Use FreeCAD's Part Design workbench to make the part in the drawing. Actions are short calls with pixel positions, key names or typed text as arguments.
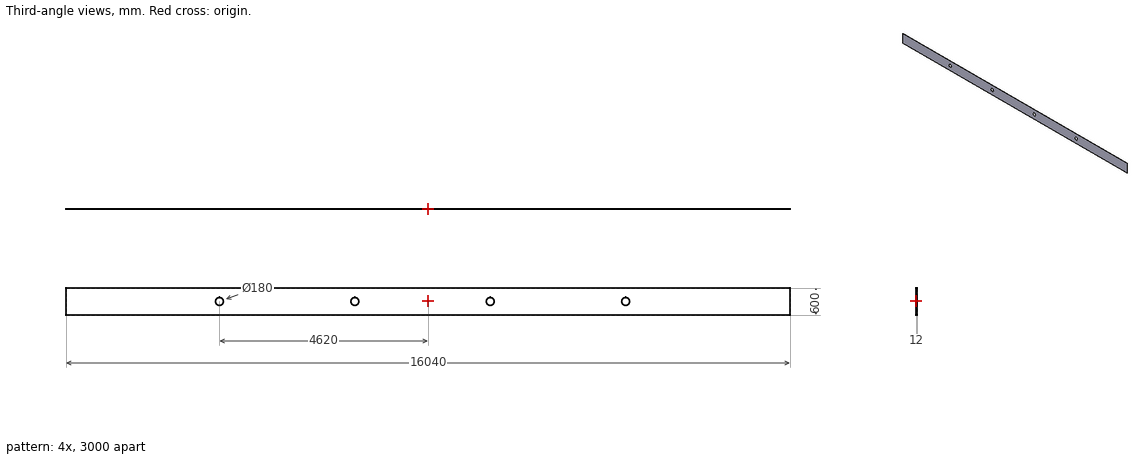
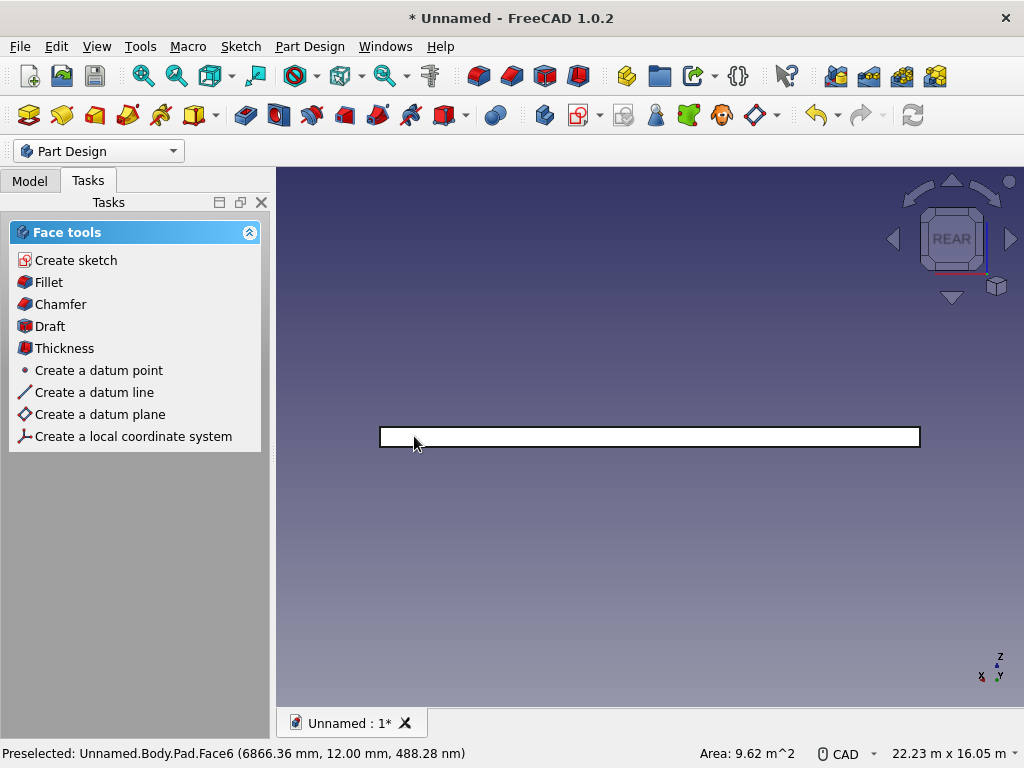
click(578, 116)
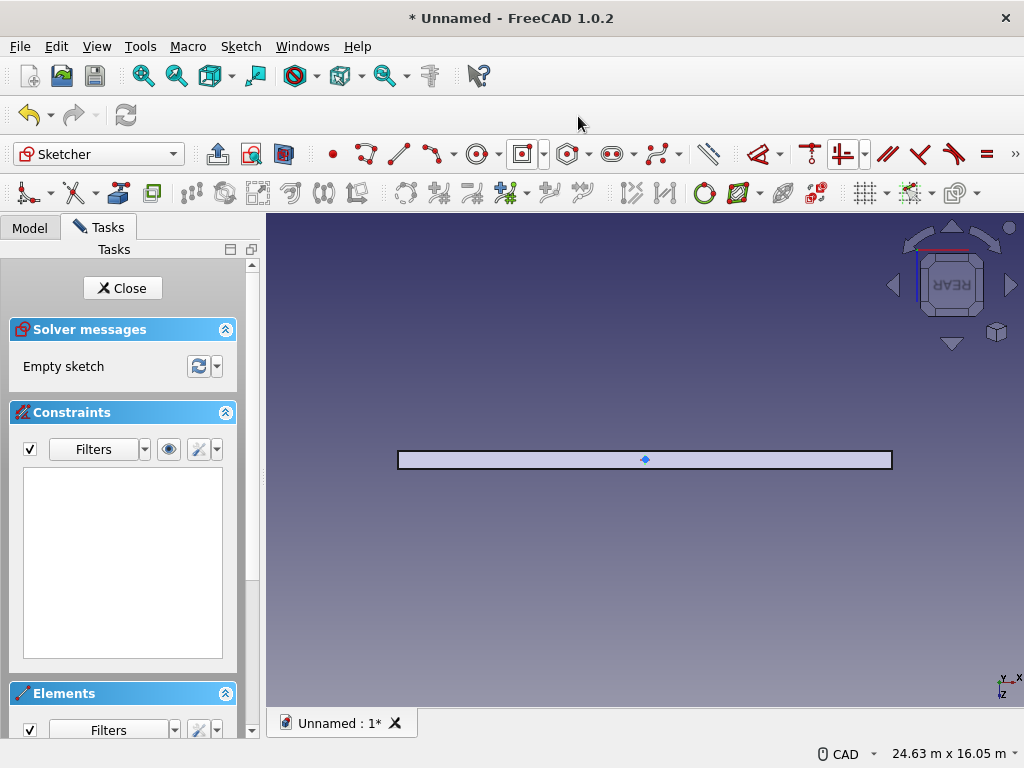
scroll(499, 460, up, 15)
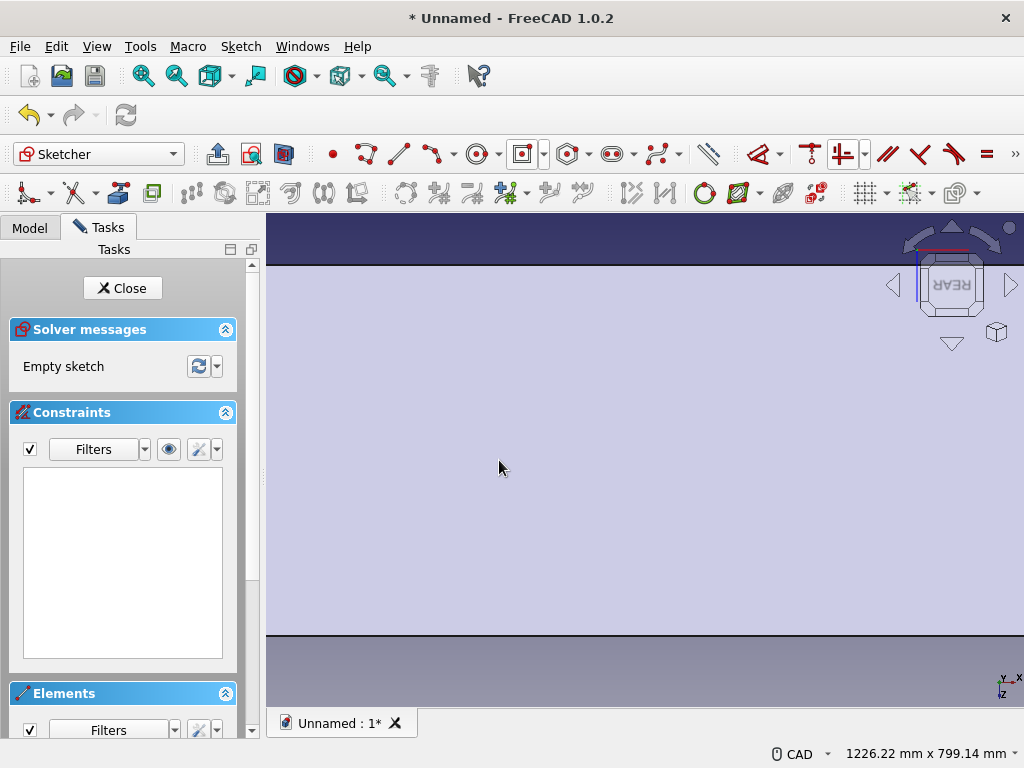
scroll(566, 445, up, 5)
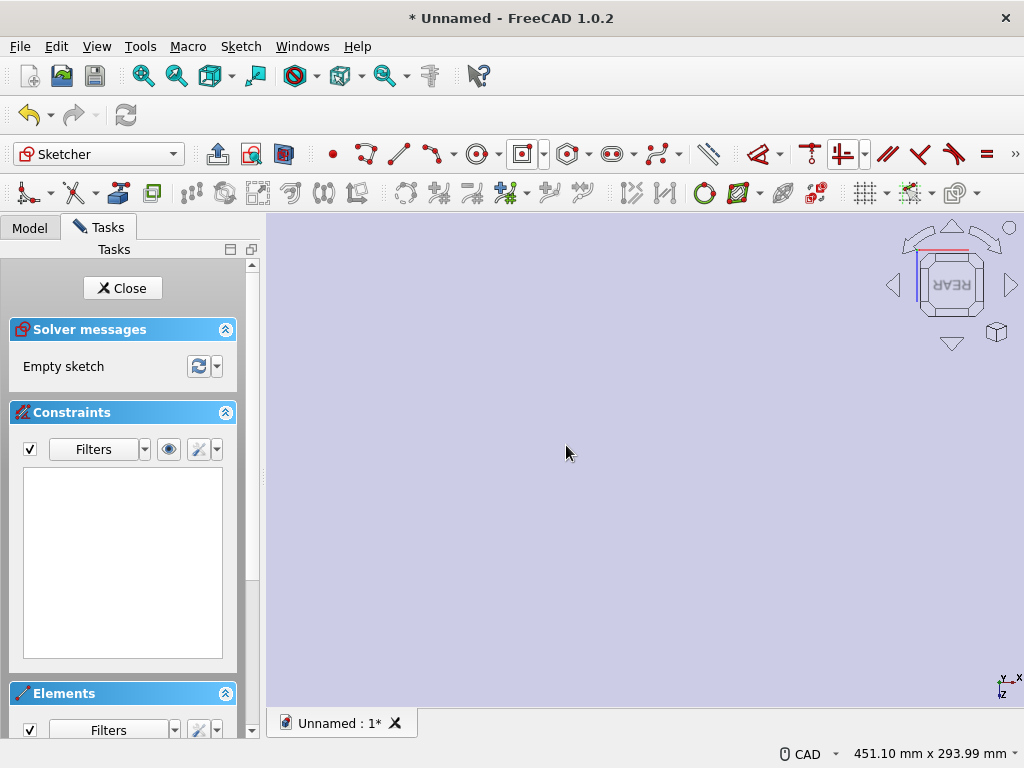
click(476, 154)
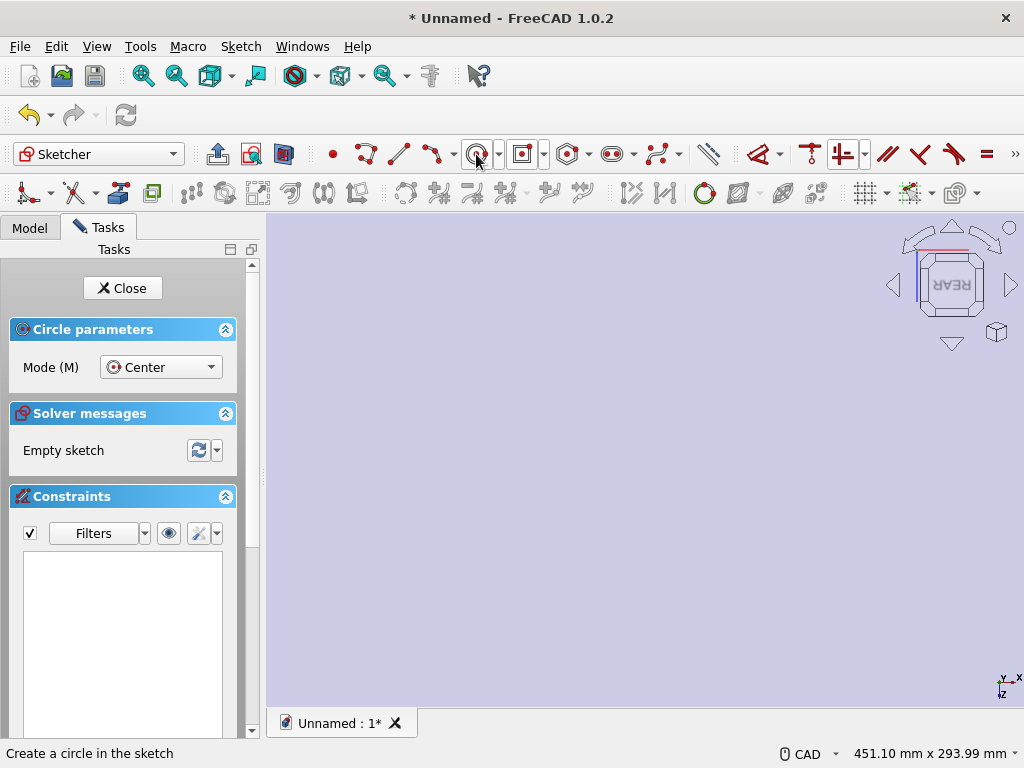
click(575, 459)
move(682, 352)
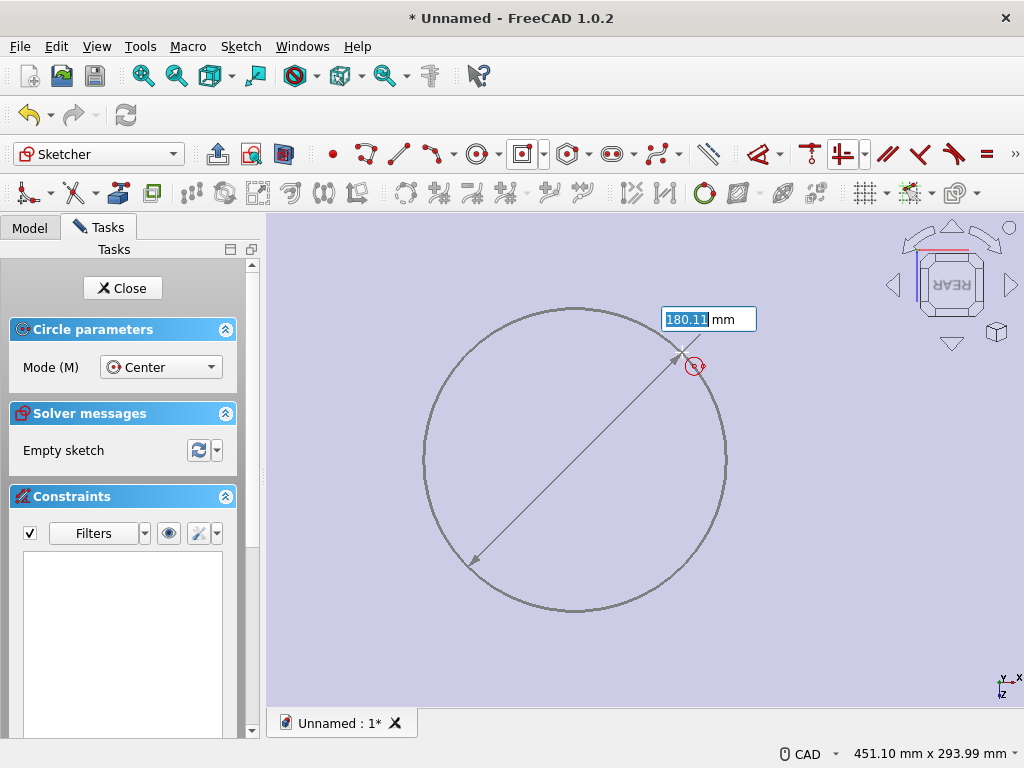
text(180)
key(Return)
key(Escape)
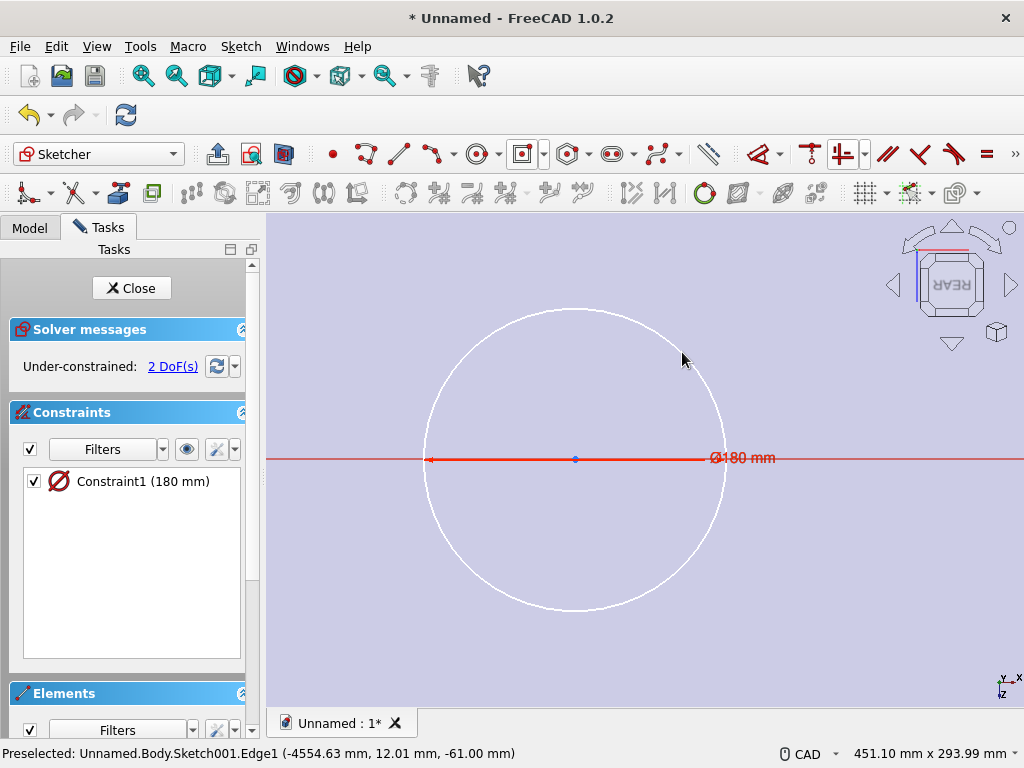
click(575, 460)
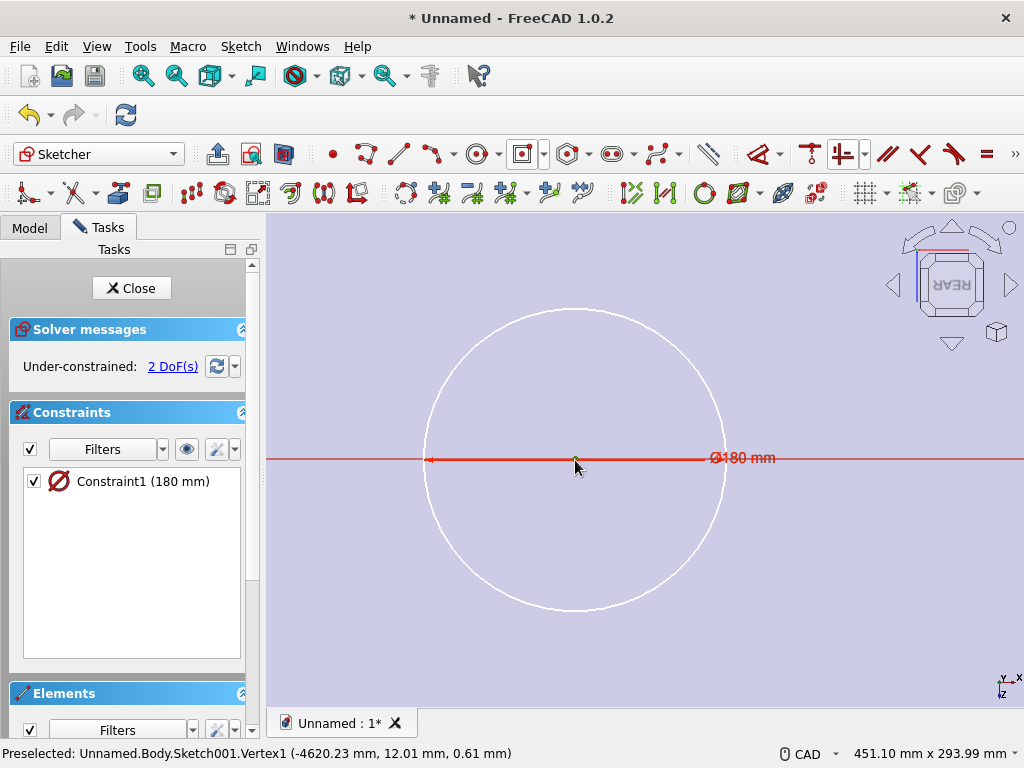
click(334, 459)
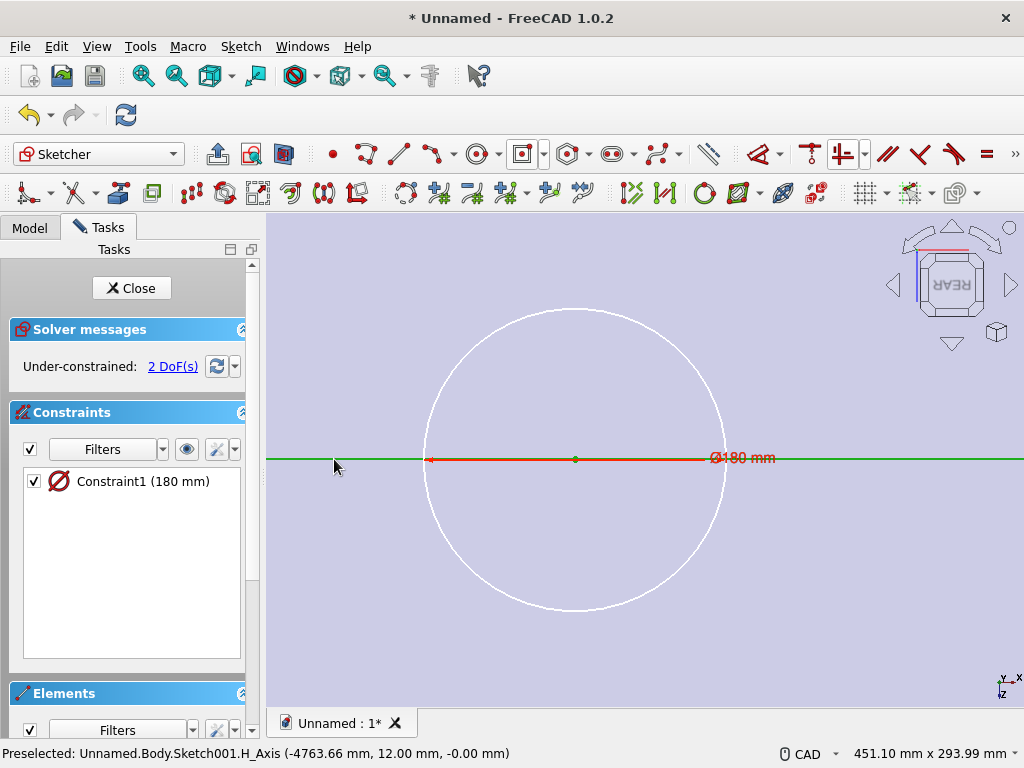
key(c)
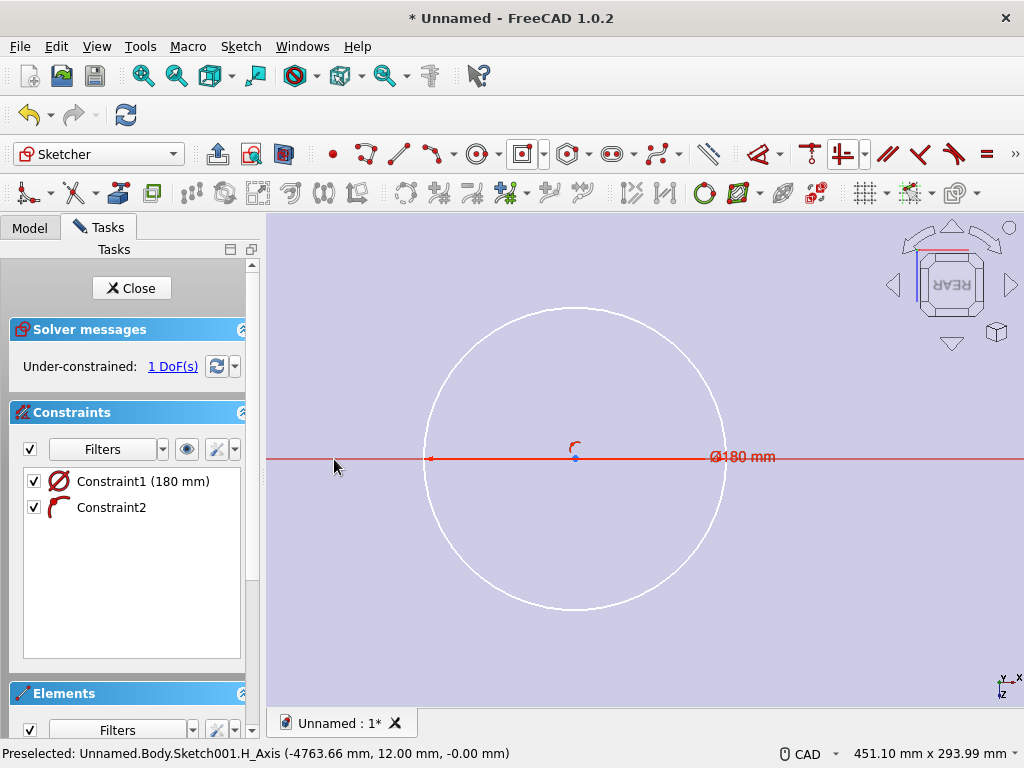
key(d)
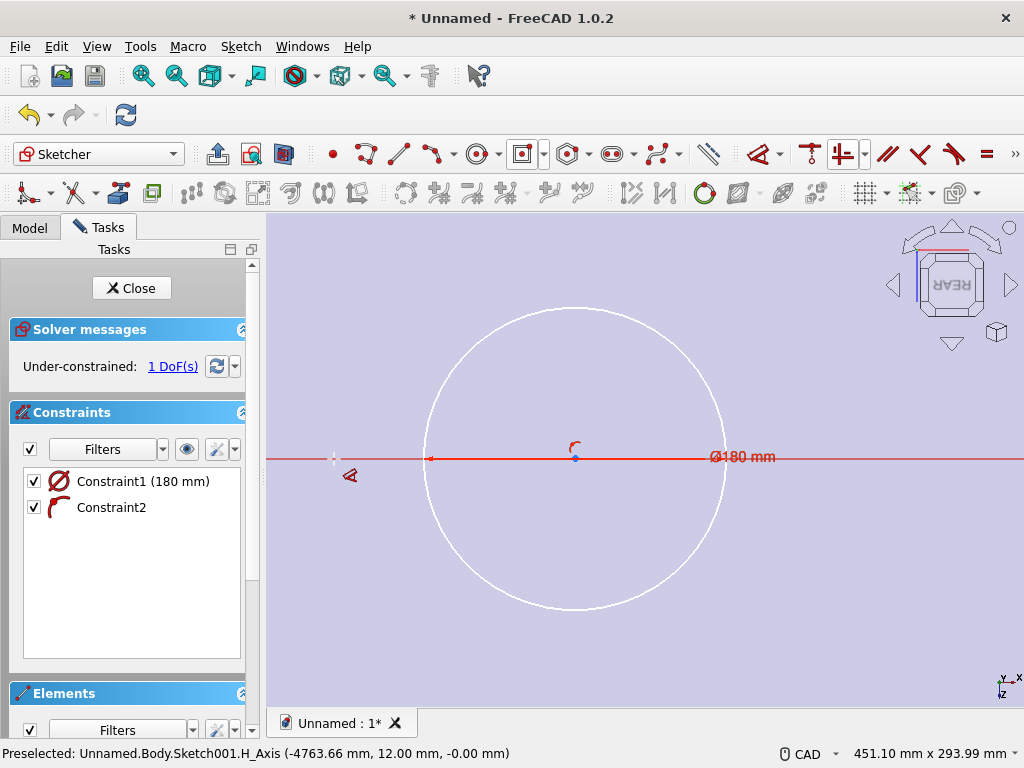
click(575, 459)
click(652, 493)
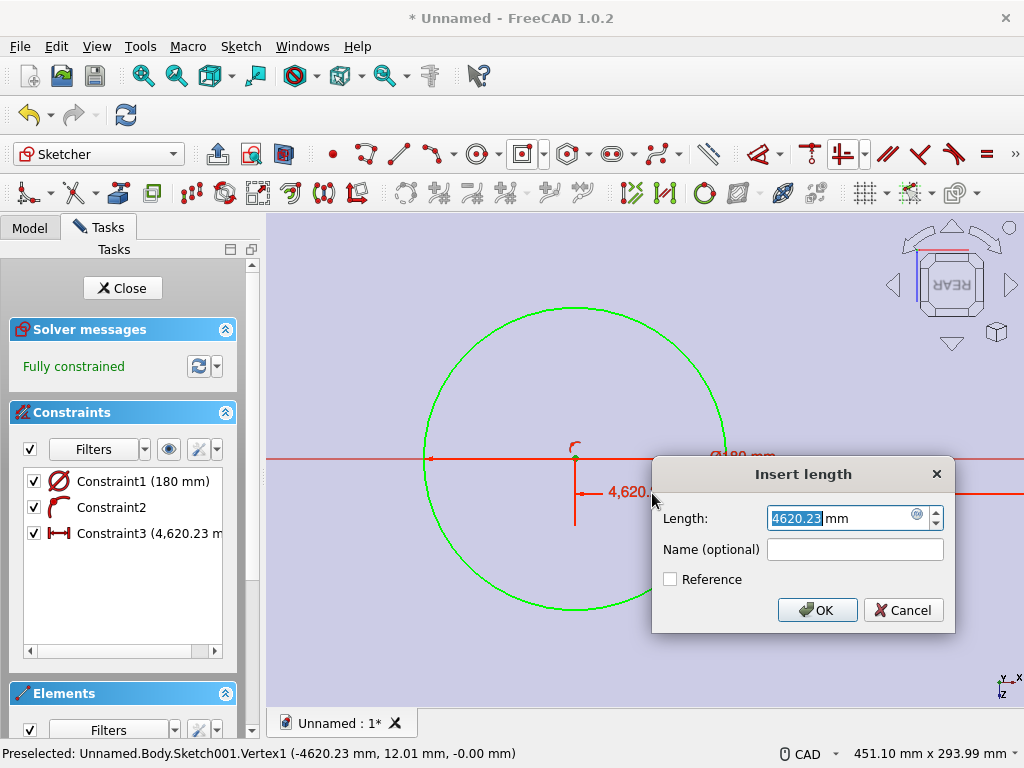
text(4620)
key(Return)
key(Escape)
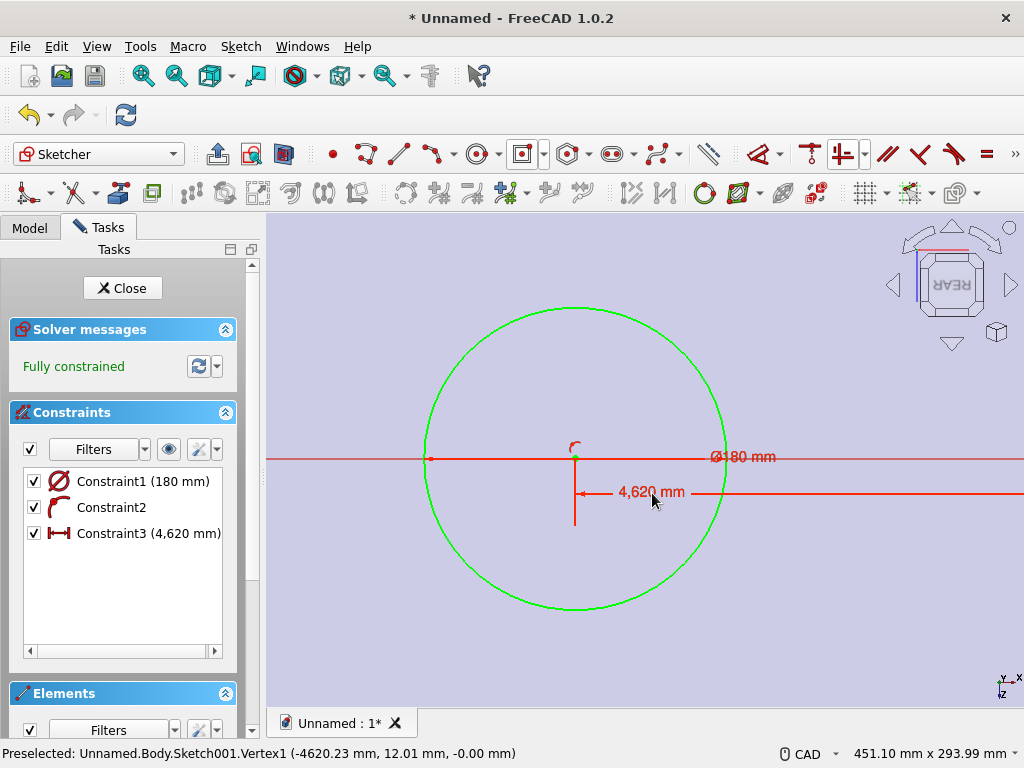
click(123, 288)